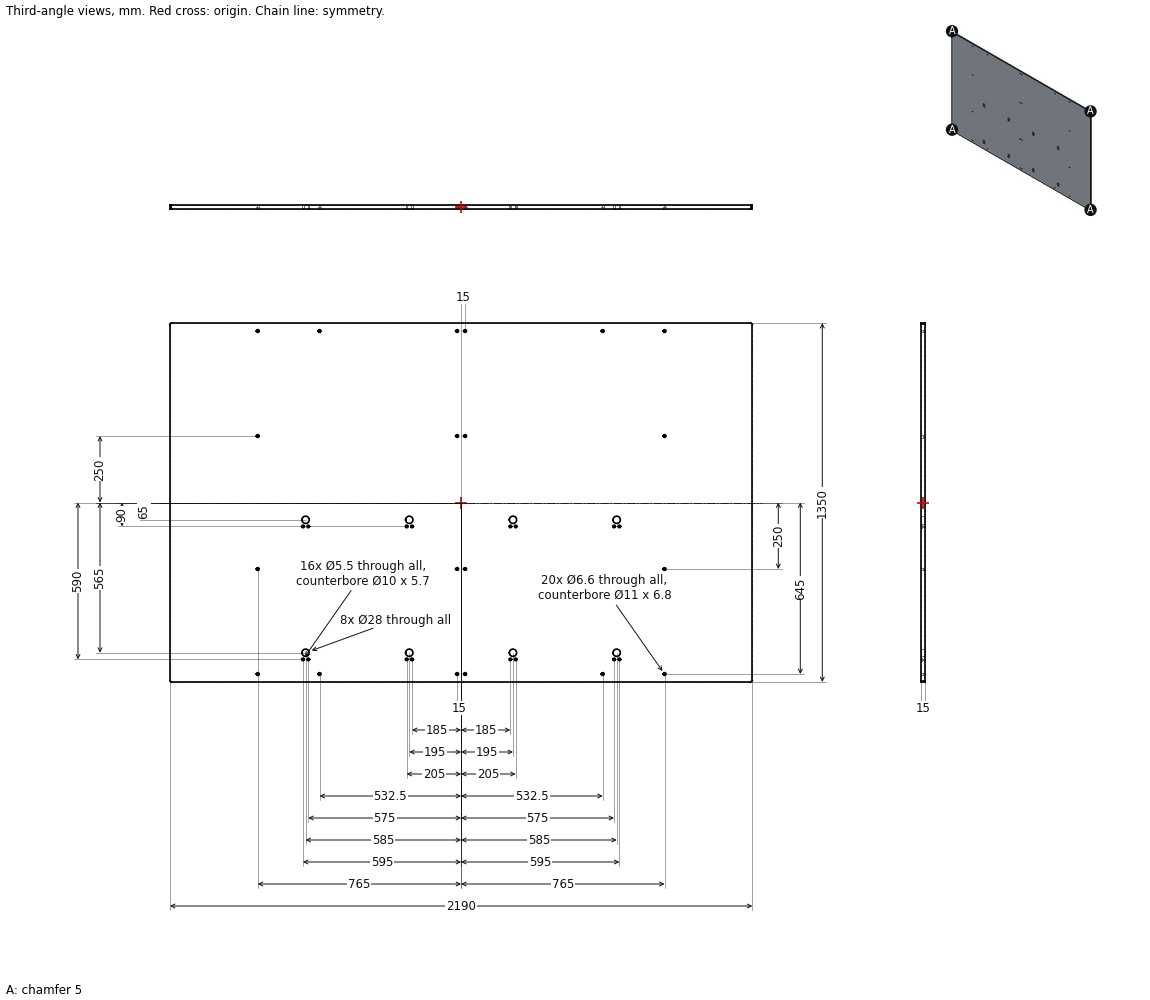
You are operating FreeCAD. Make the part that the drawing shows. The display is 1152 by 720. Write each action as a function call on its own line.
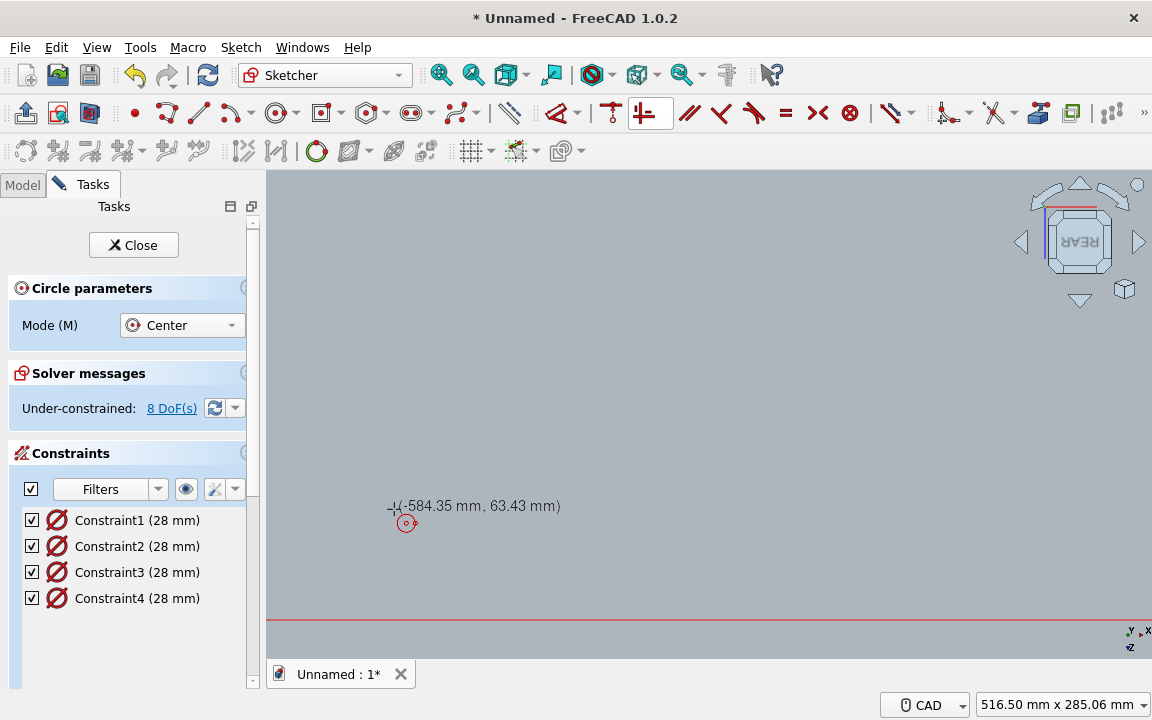
scroll(393, 510, down, 7)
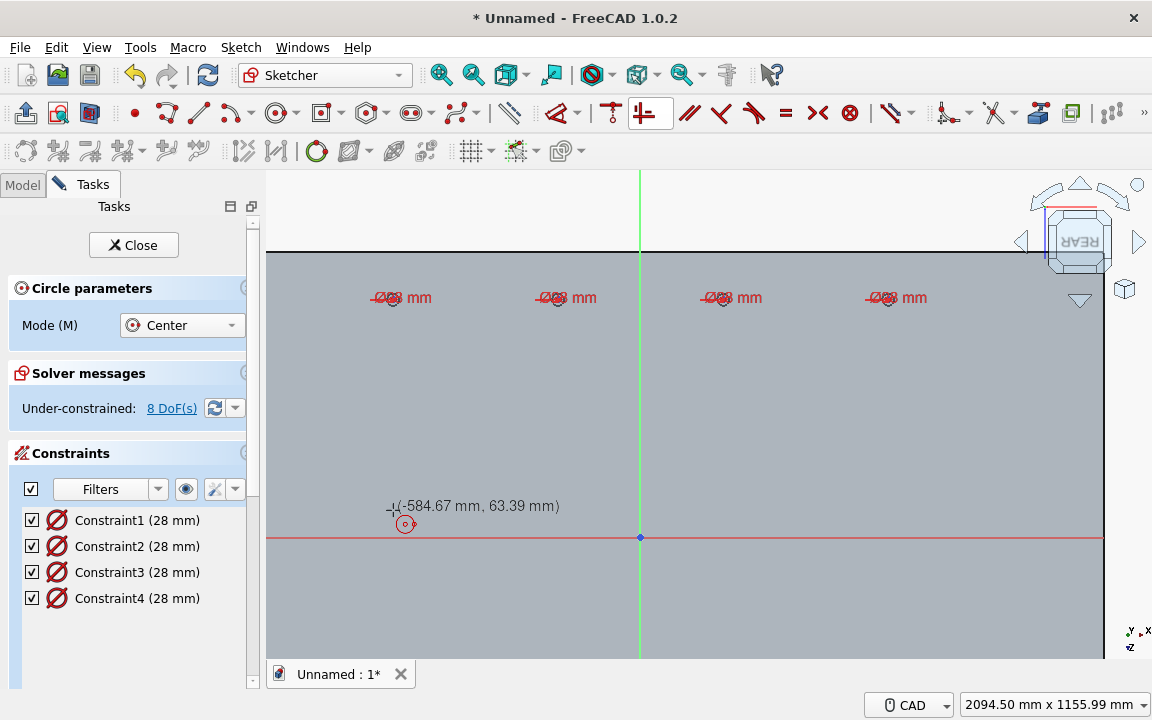
click(393, 510)
move(397, 506)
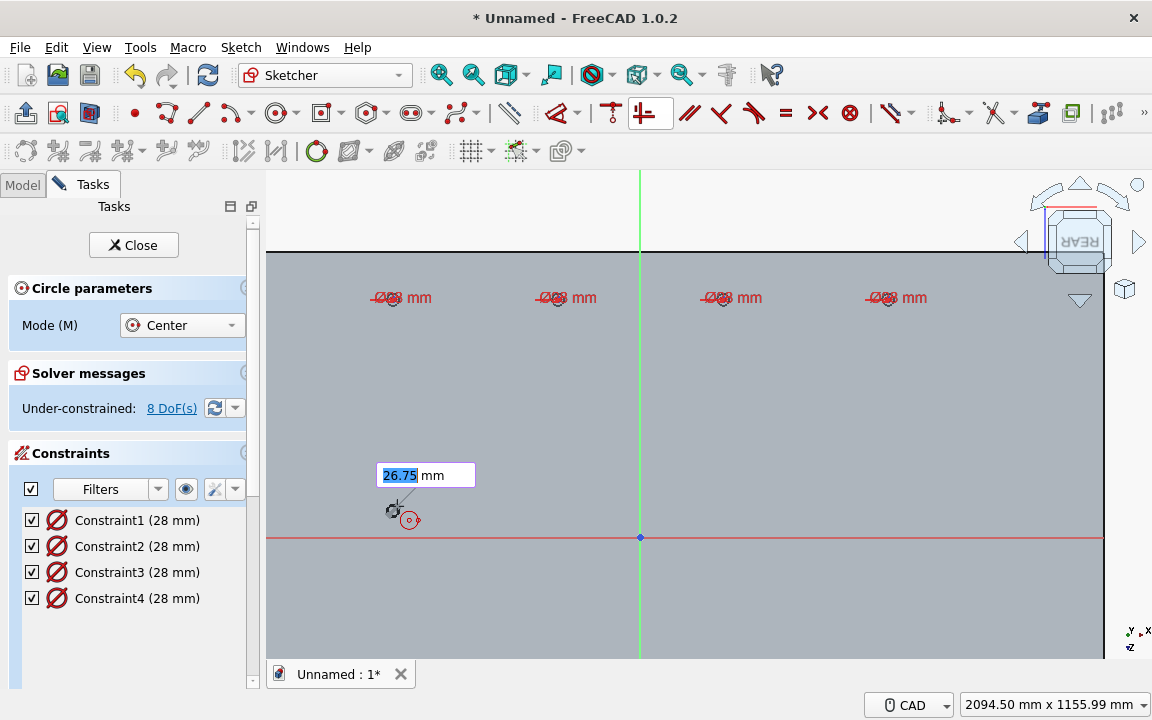
text(28)
key(Return)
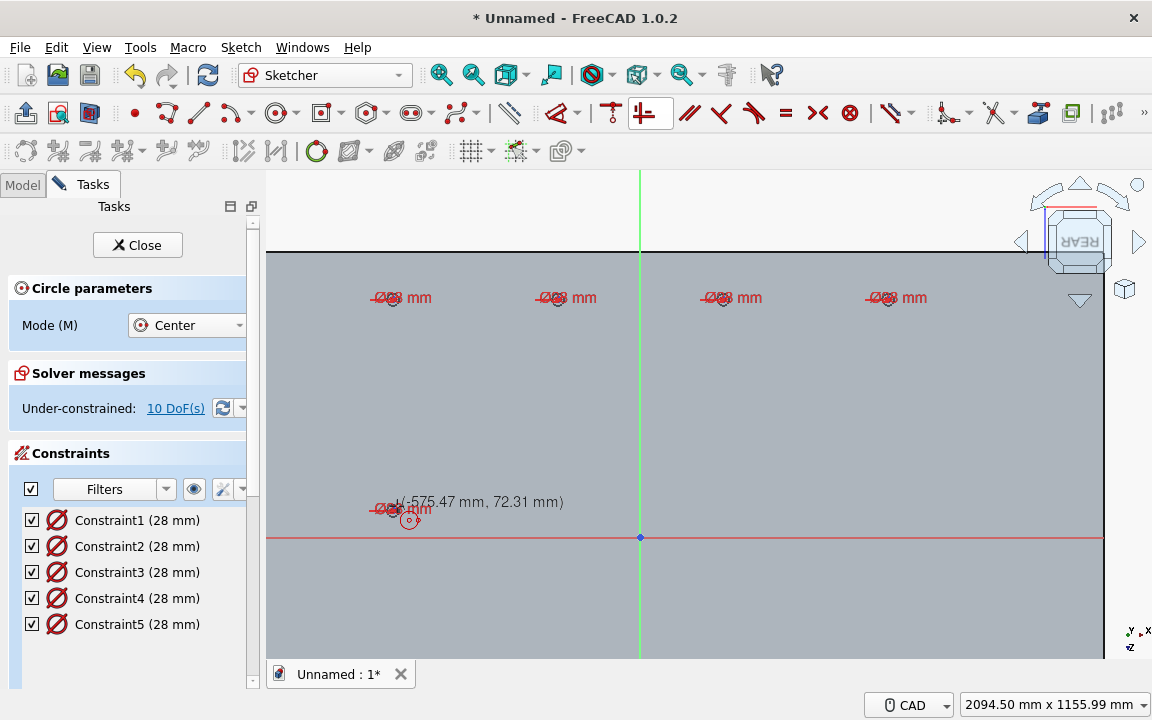
scroll(558, 510, up, 7)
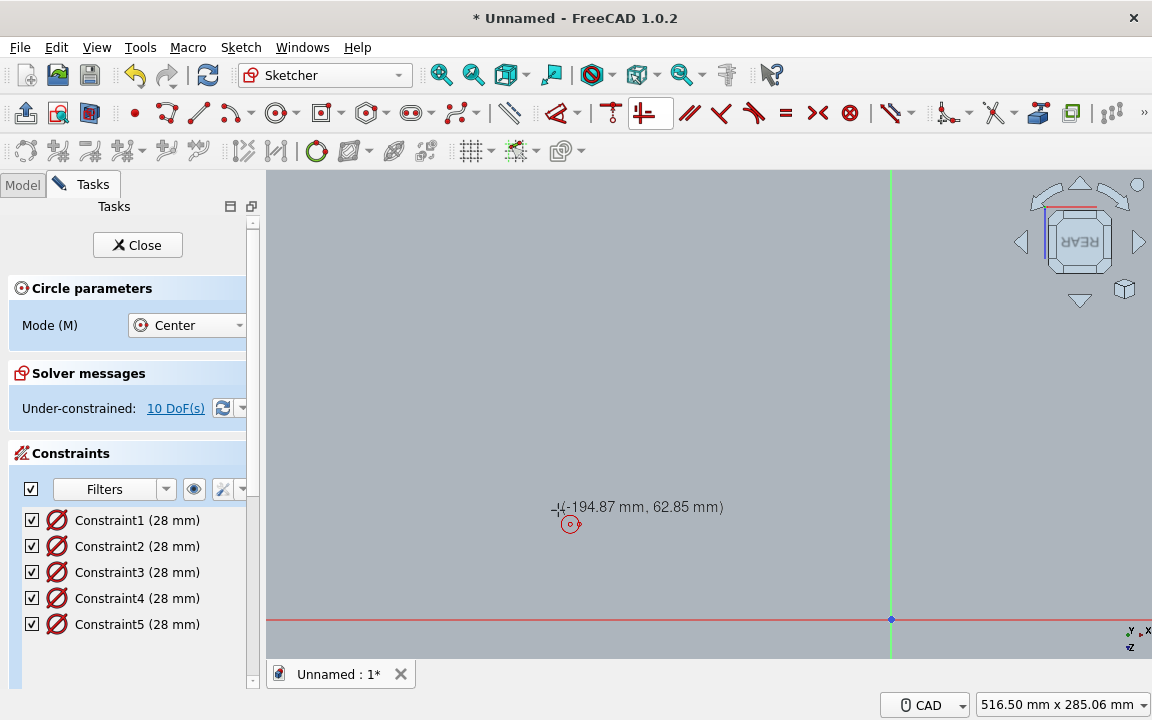
scroll(558, 510, down, 7)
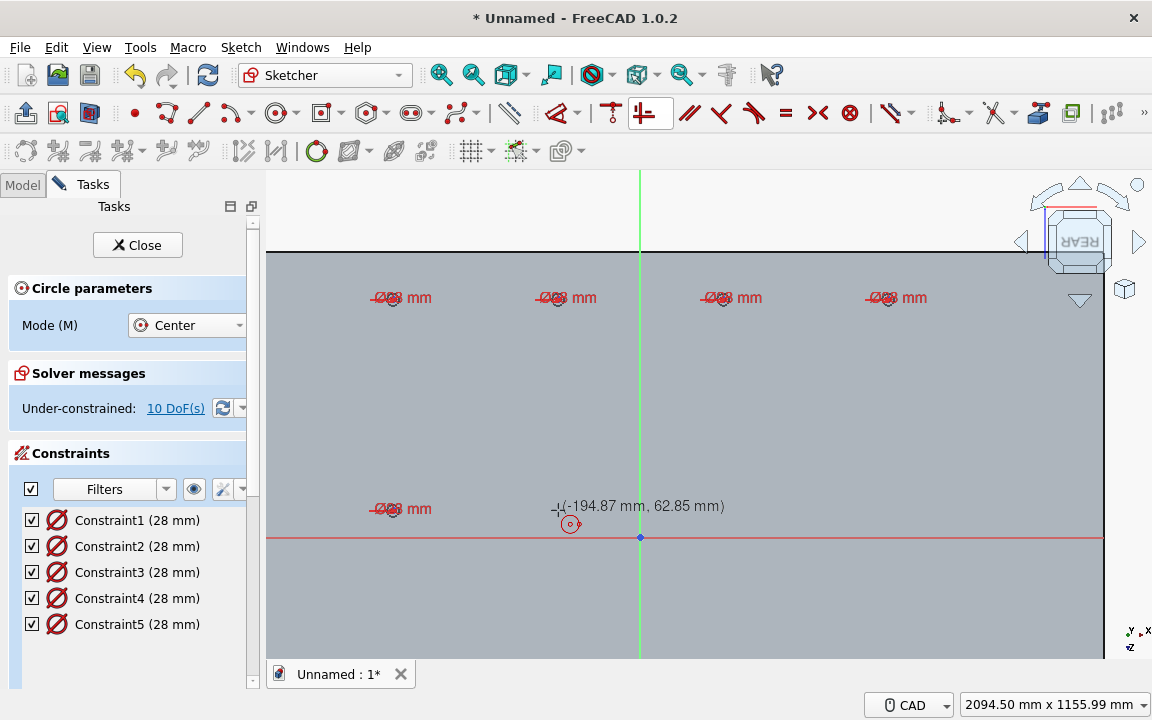
click(558, 510)
move(562, 506)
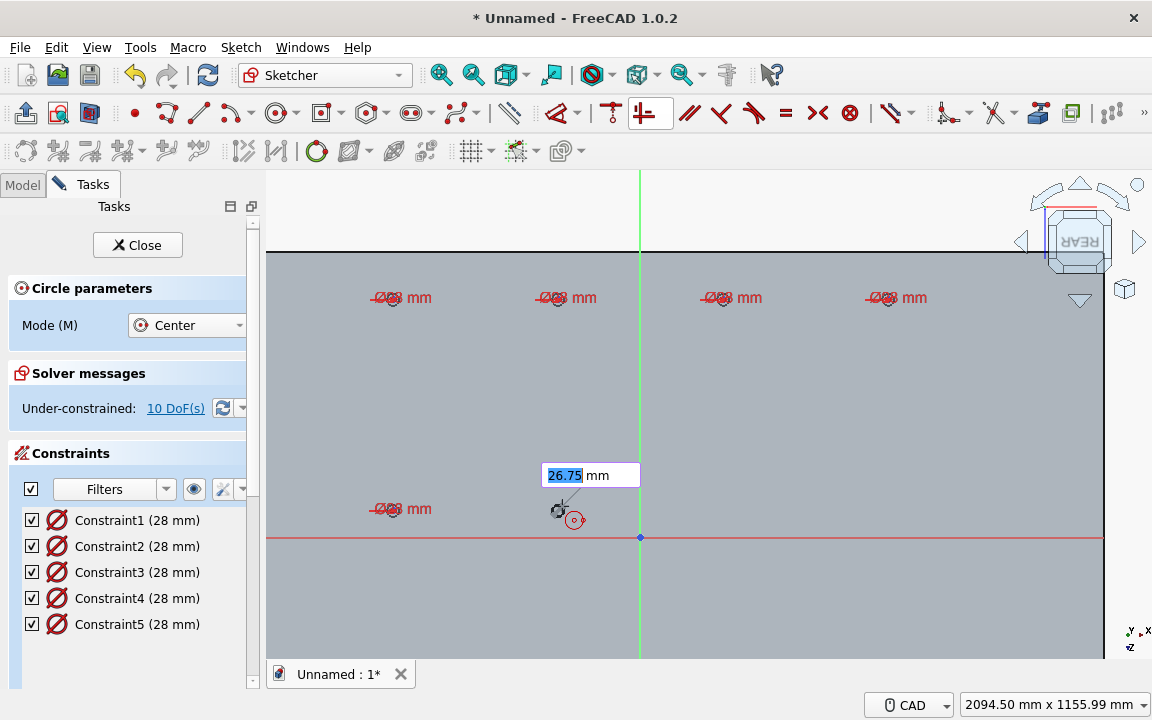
text(28)
key(Return)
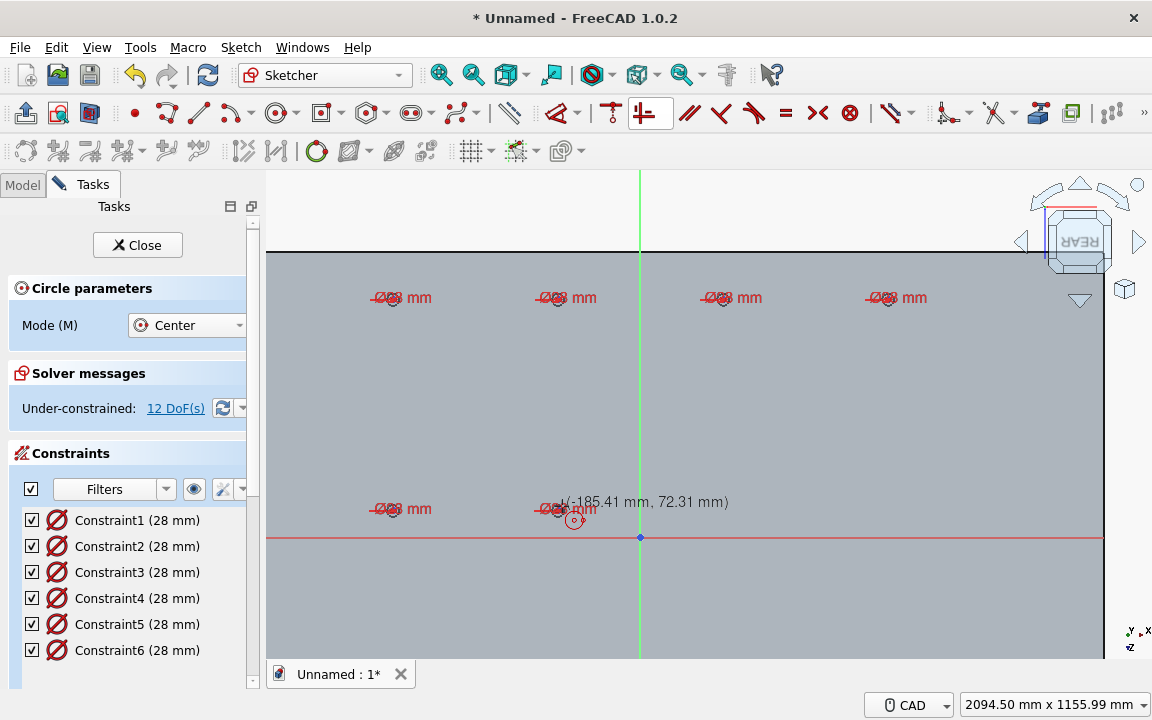
scroll(723, 510, up, 7)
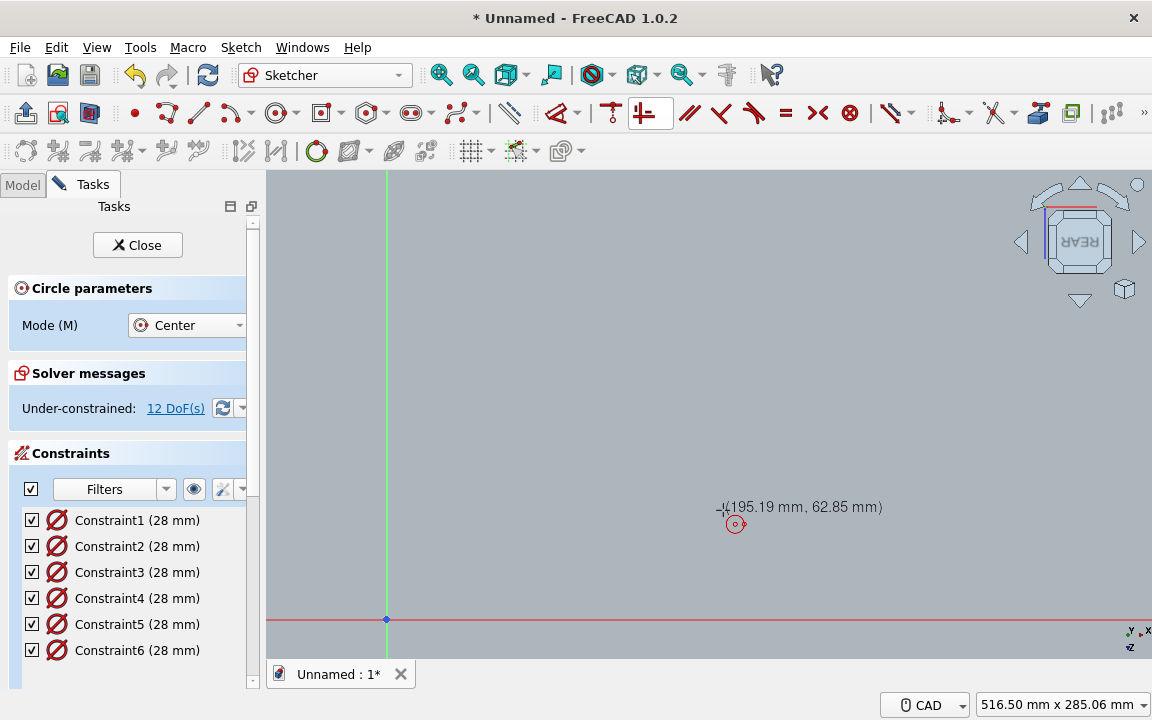
scroll(724, 510, down, 7)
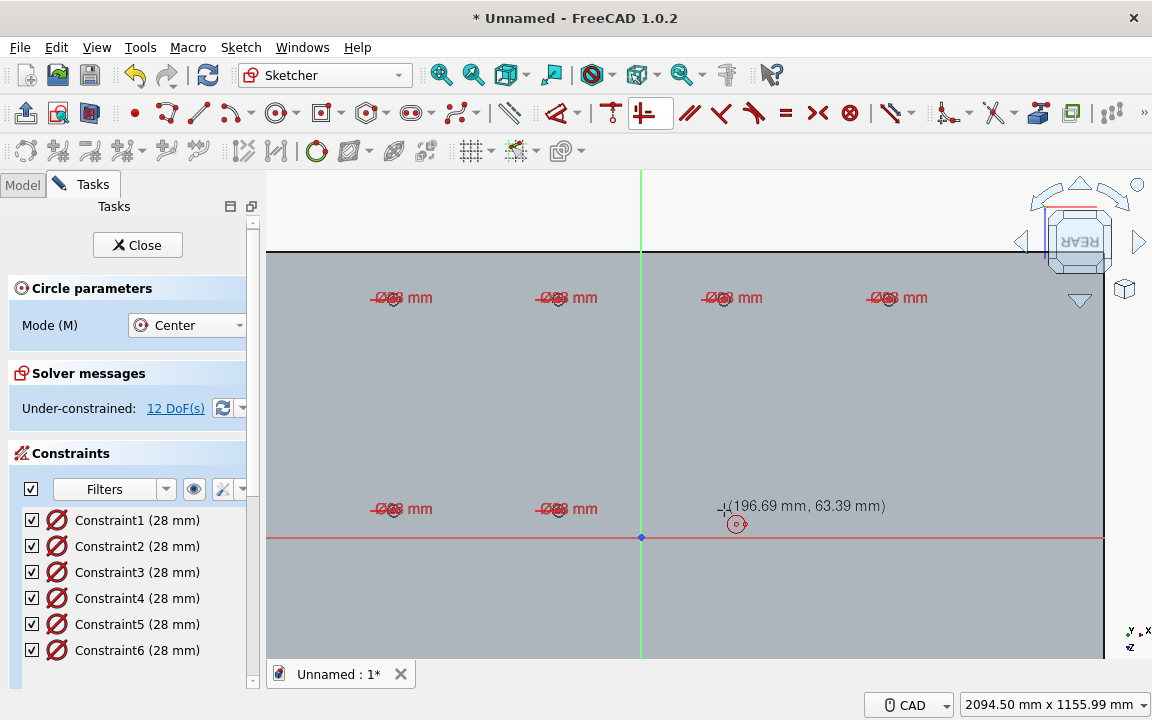
click(724, 510)
move(728, 506)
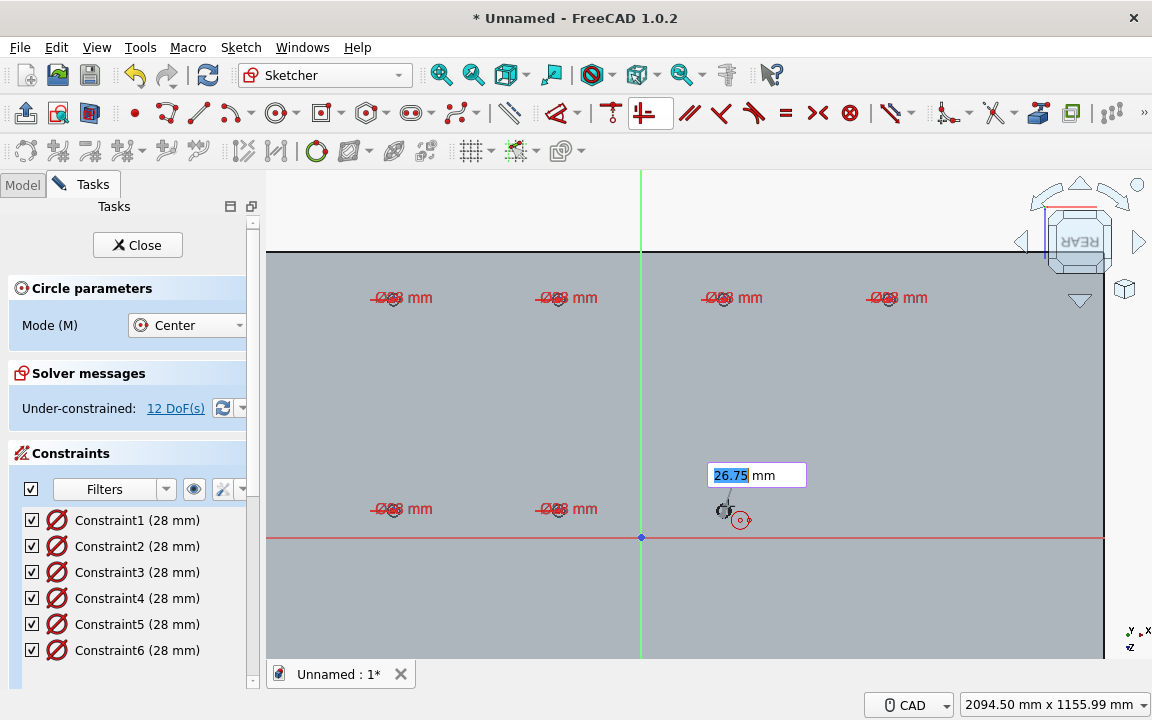
text(28)
key(Return)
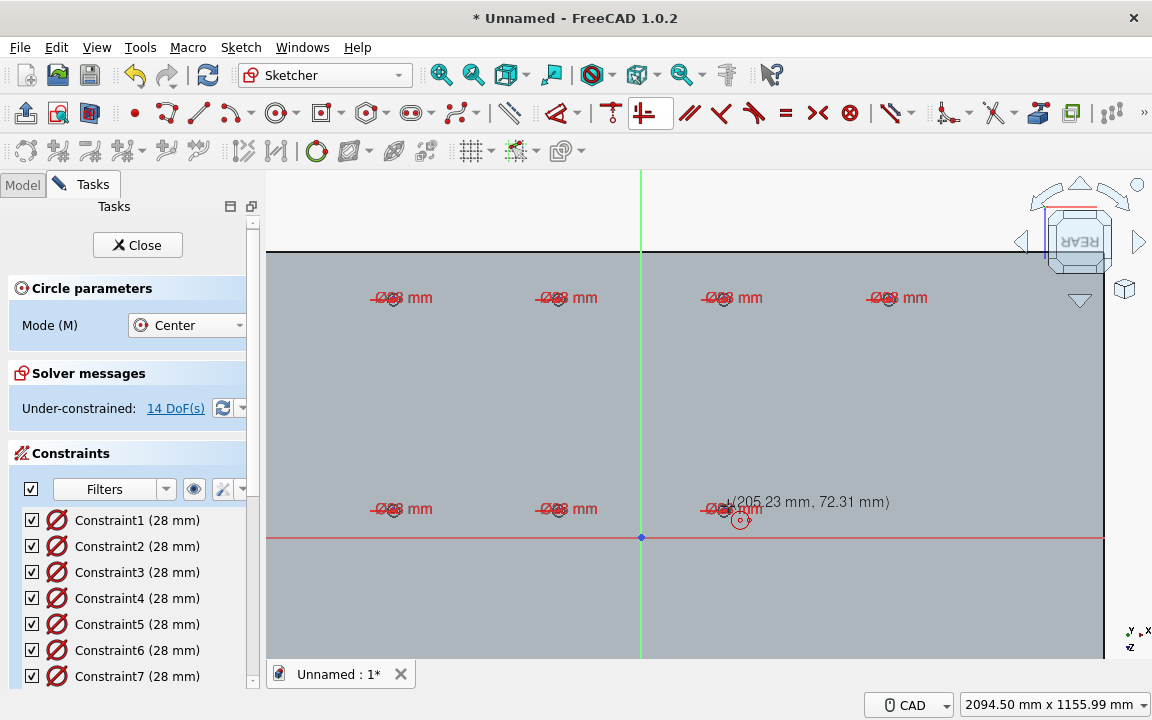
scroll(889, 510, up, 7)